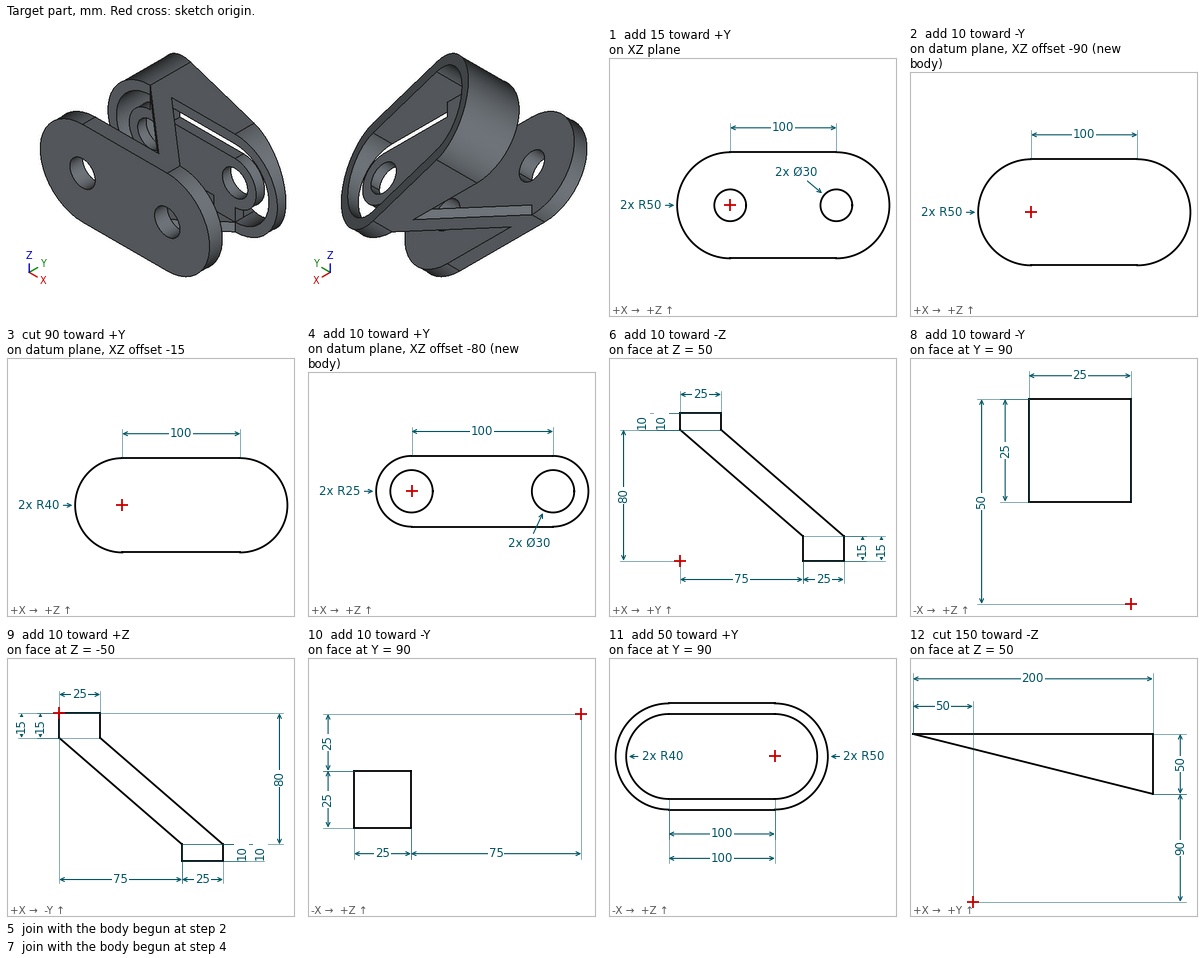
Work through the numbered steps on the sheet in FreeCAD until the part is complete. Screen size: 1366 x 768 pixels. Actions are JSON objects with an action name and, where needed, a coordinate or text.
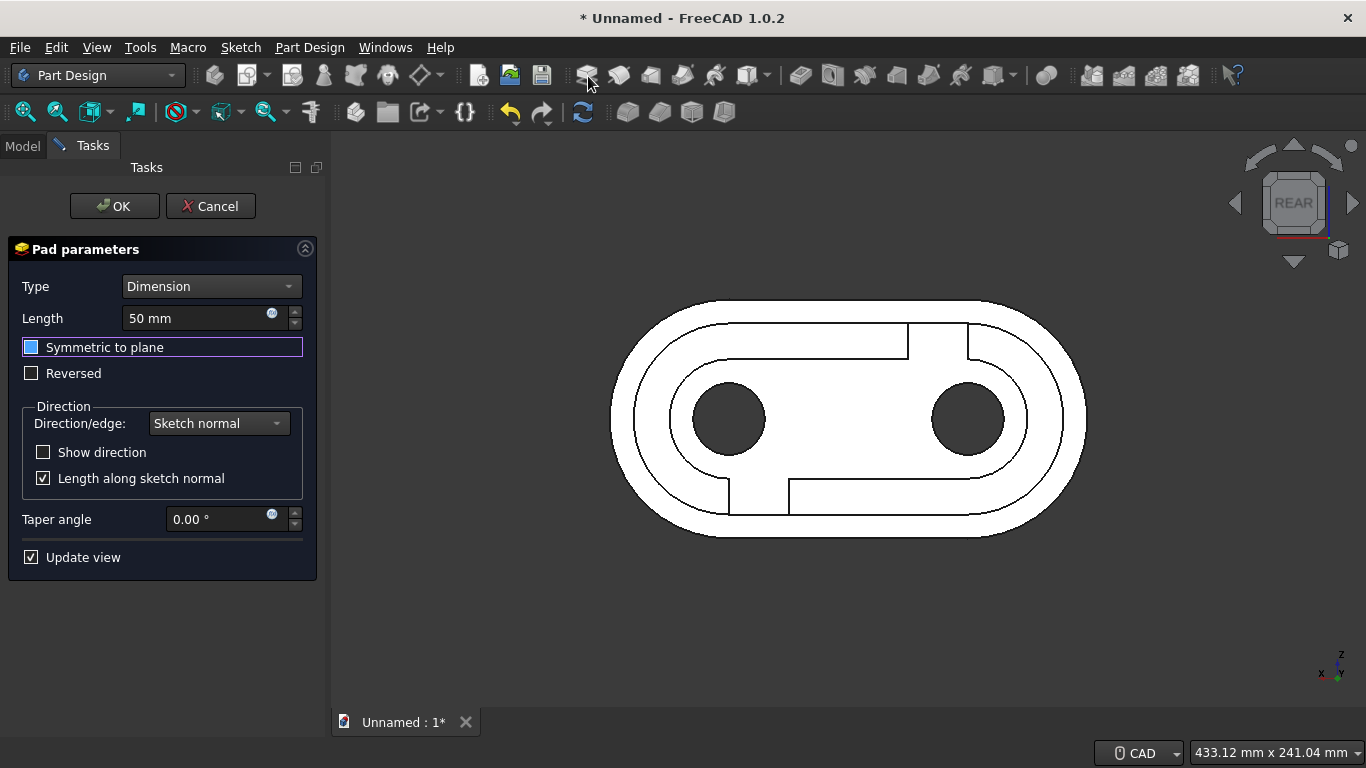
{"action": "left_click", "coordinate": [115, 206]}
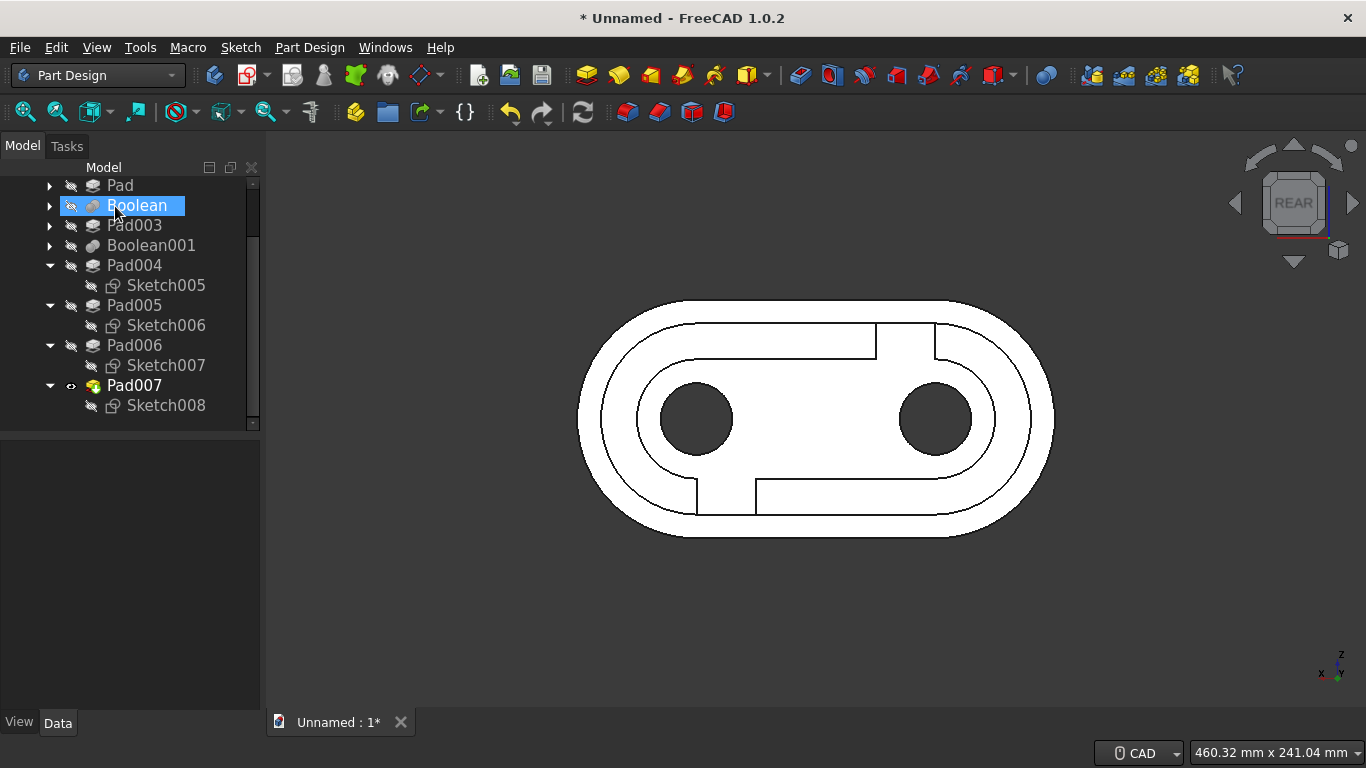
{"action": "left_click", "coordinate": [26, 112]}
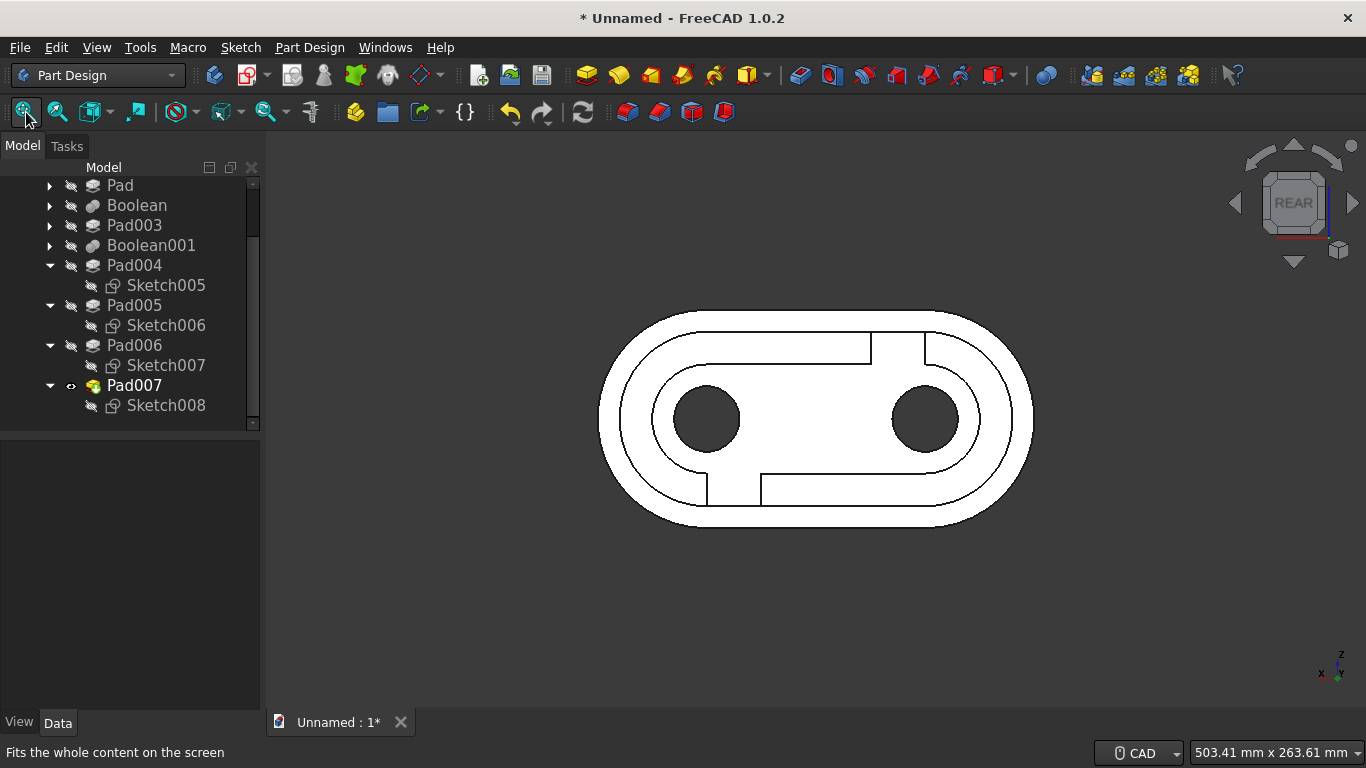
{"action": "key", "text": "0"}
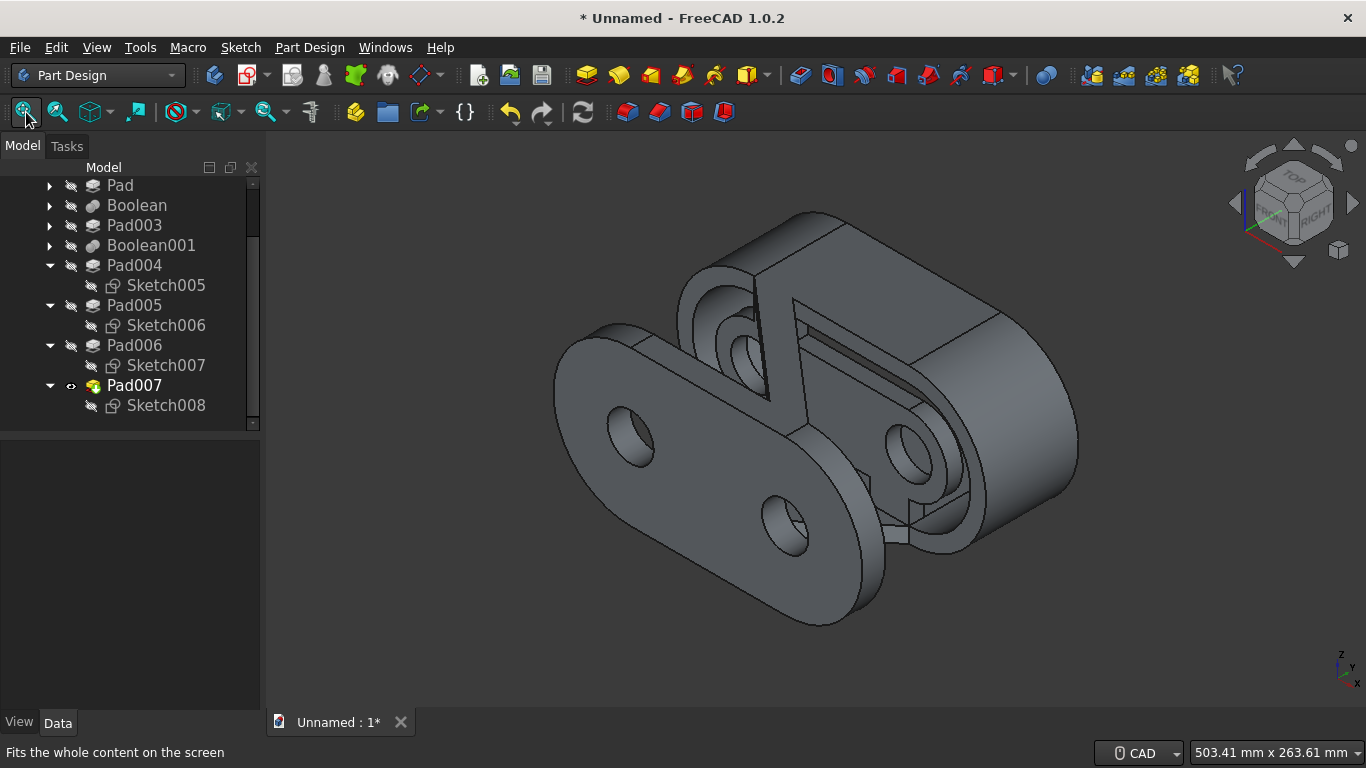
{"action": "left_click", "coordinate": [900, 306]}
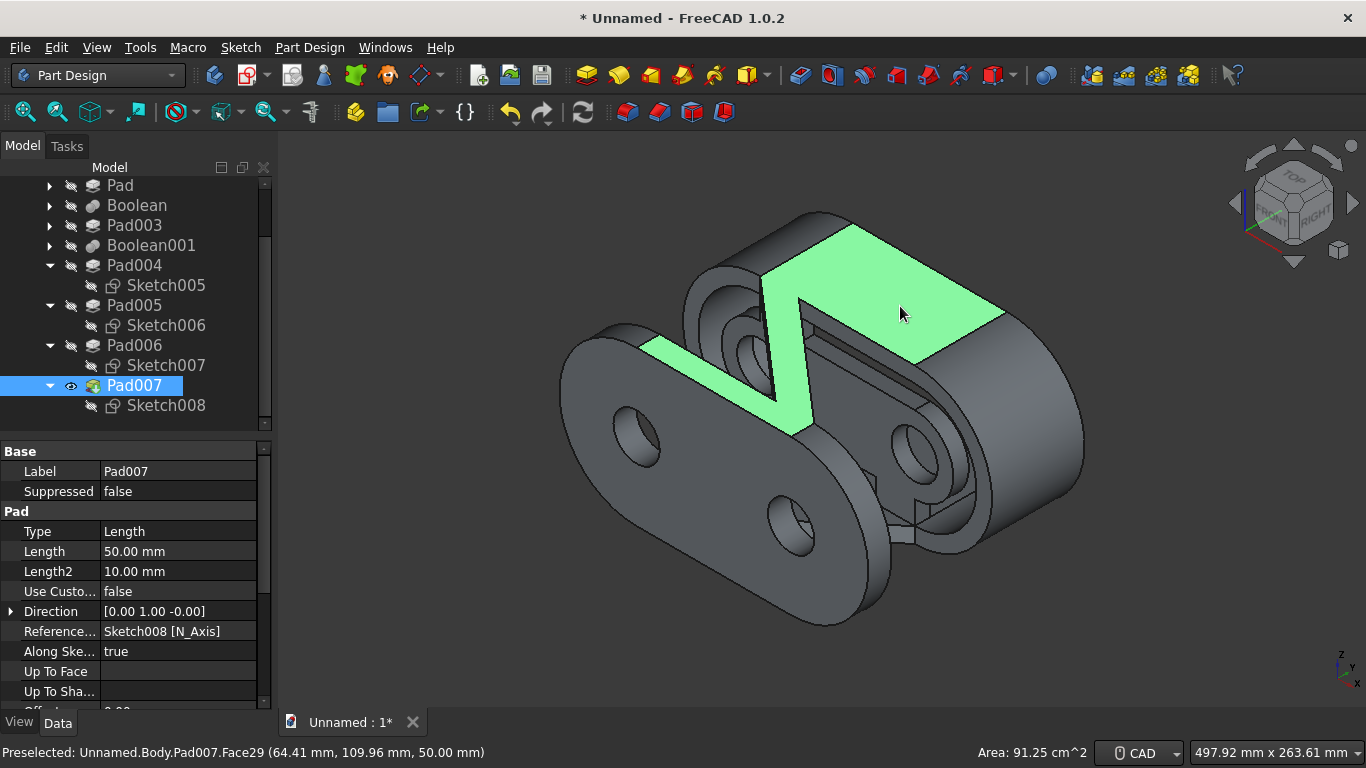
{"action": "left_click", "coordinate": [248, 76]}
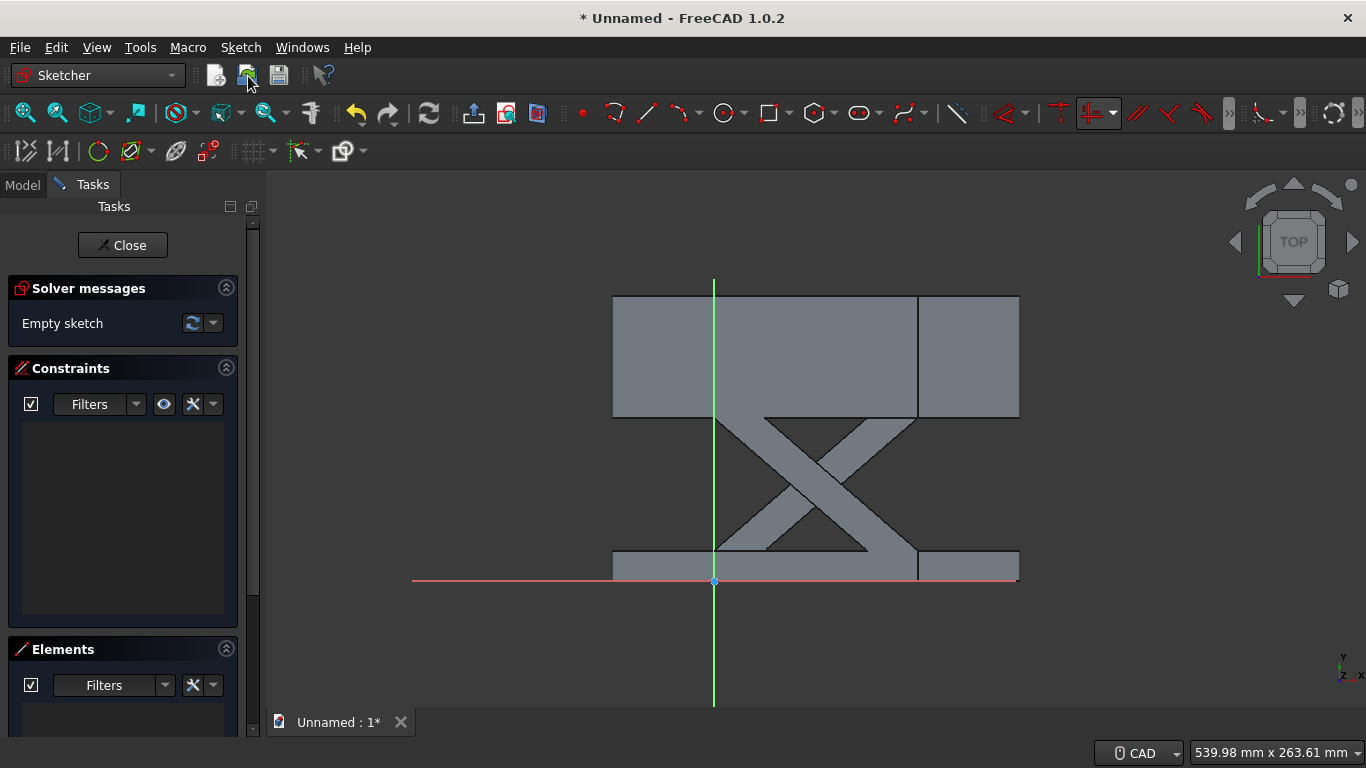
{"action": "left_click", "coordinate": [616, 114]}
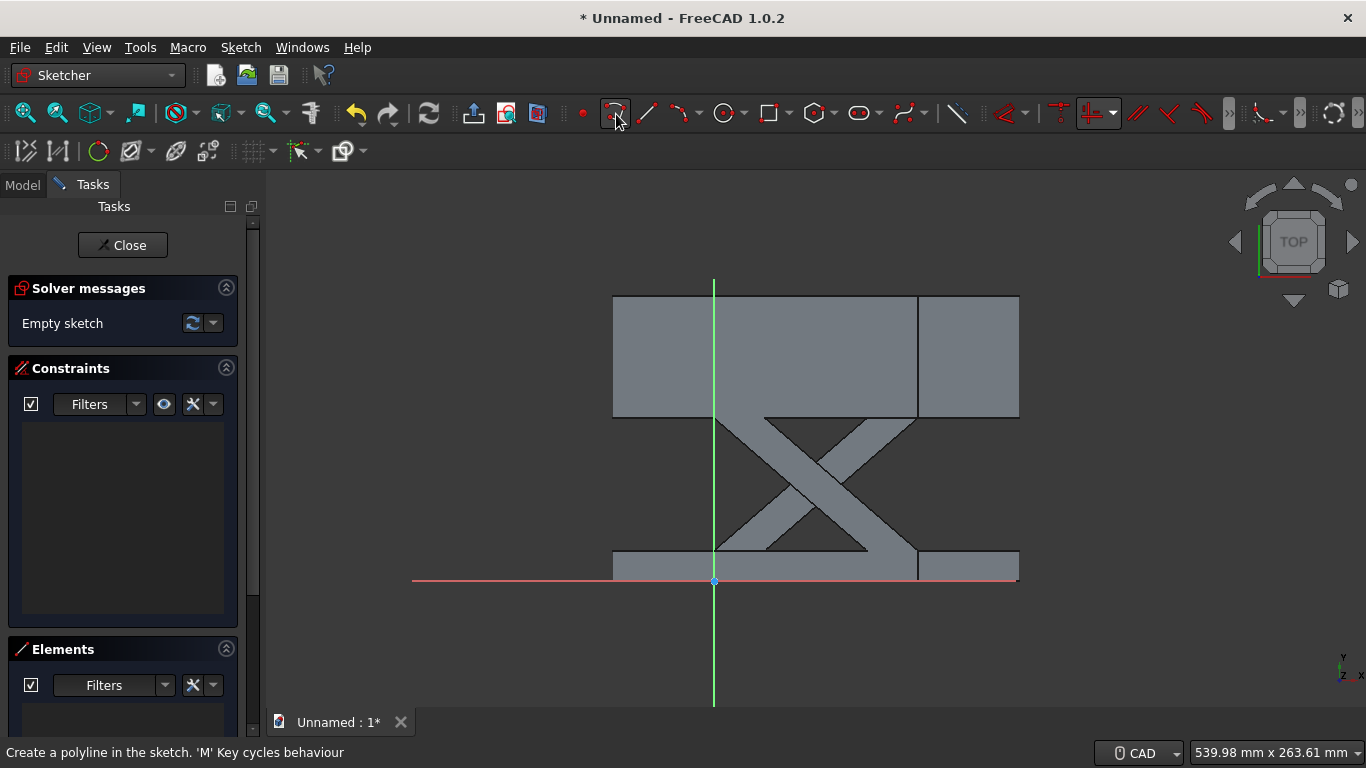
{"action": "left_click", "coordinate": [612, 296]}
{"action": "left_click", "coordinate": [1020, 398]}
{"action": "left_click", "coordinate": [1020, 296]}
{"action": "left_click", "coordinate": [612, 297]}
{"action": "key", "text": "Escape"}
{"action": "key", "text": "Escape"}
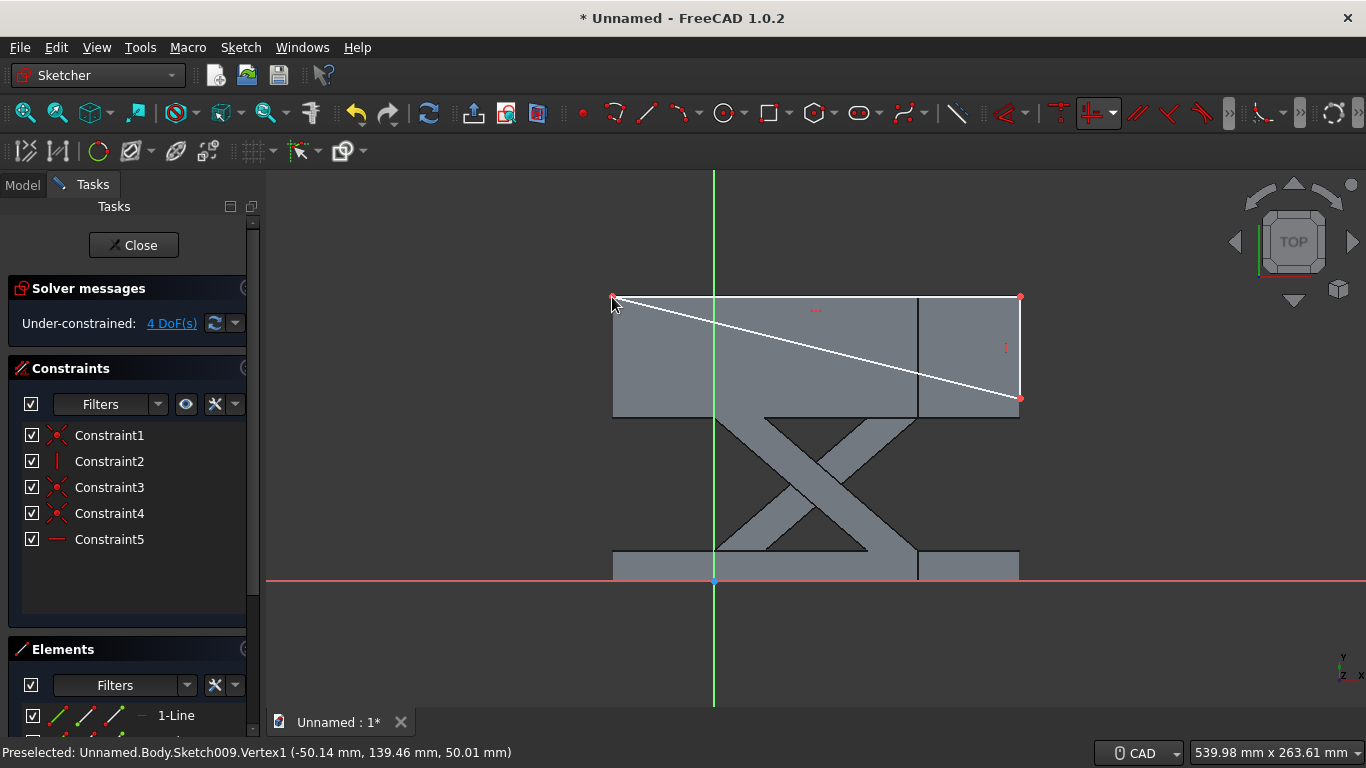
{"action": "left_click", "coordinate": [1004, 114]}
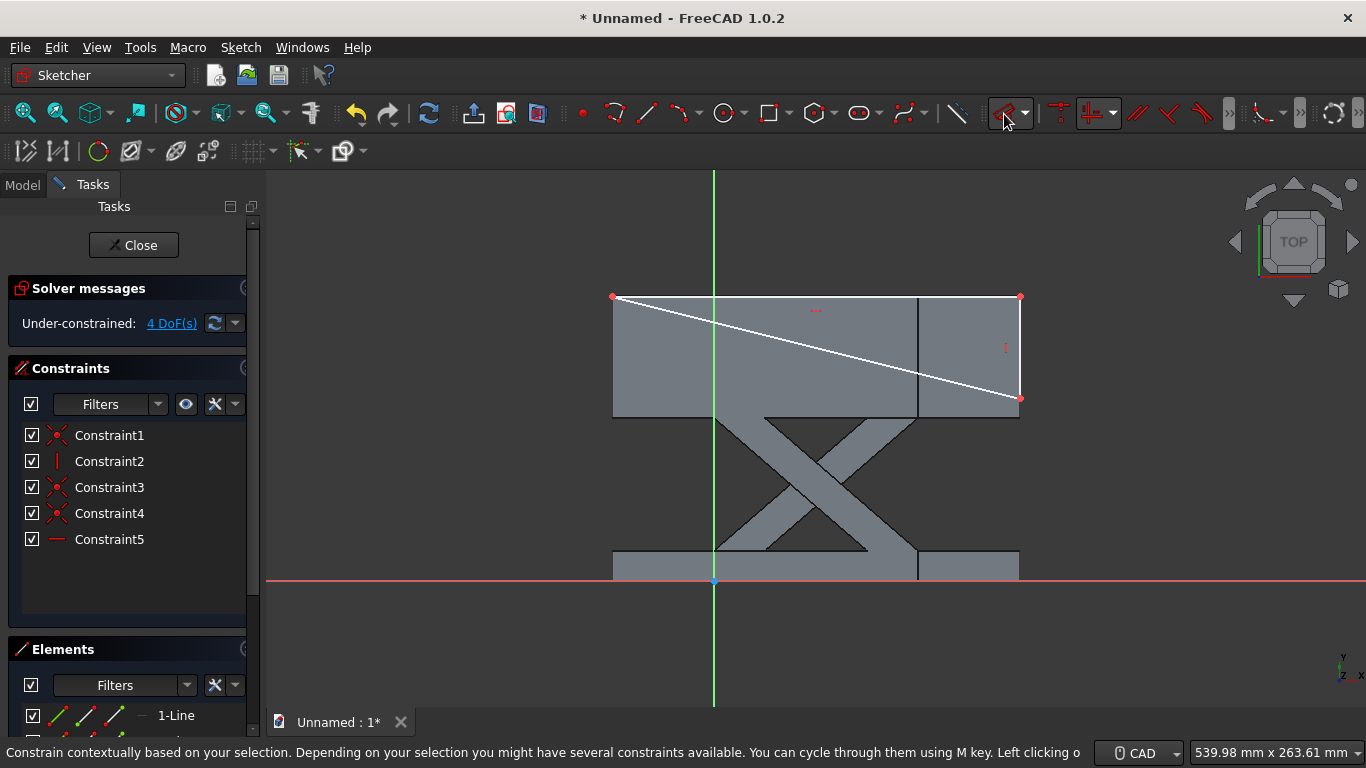
{"action": "left_click", "coordinate": [1020, 368]}
{"action": "left_click", "coordinate": [1054, 348]}